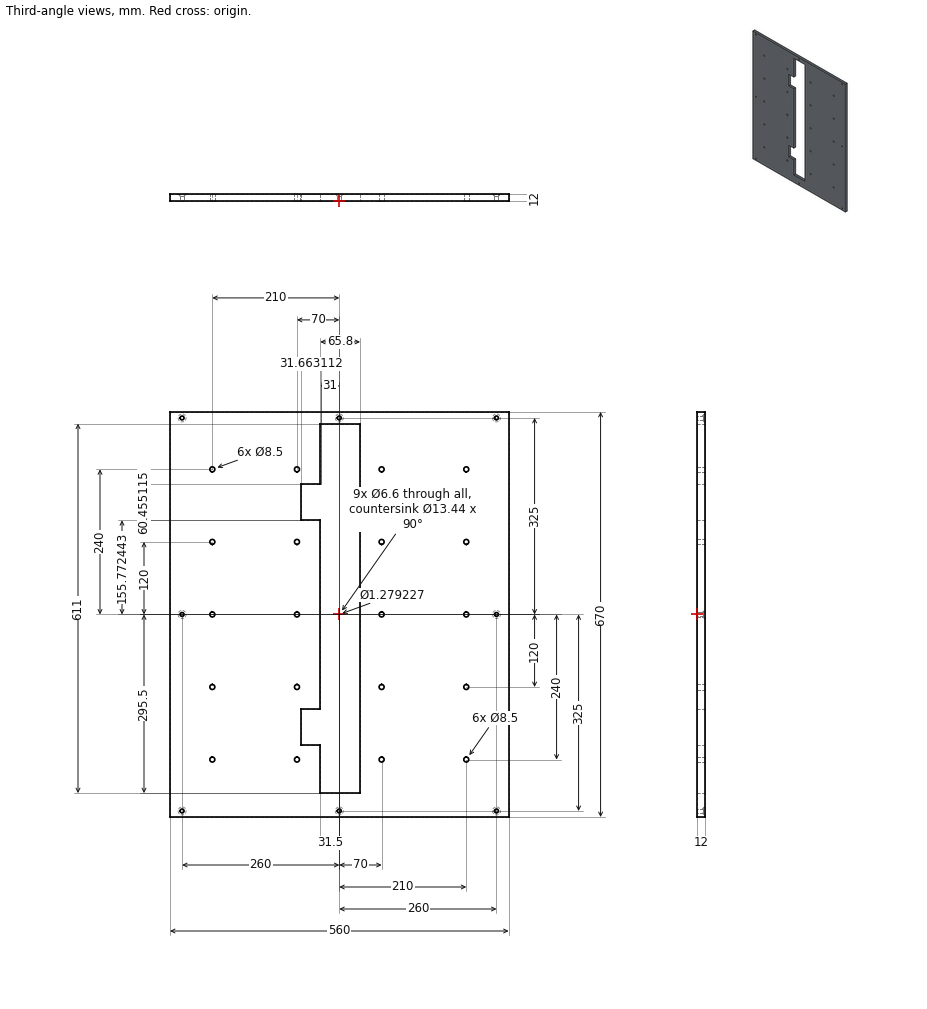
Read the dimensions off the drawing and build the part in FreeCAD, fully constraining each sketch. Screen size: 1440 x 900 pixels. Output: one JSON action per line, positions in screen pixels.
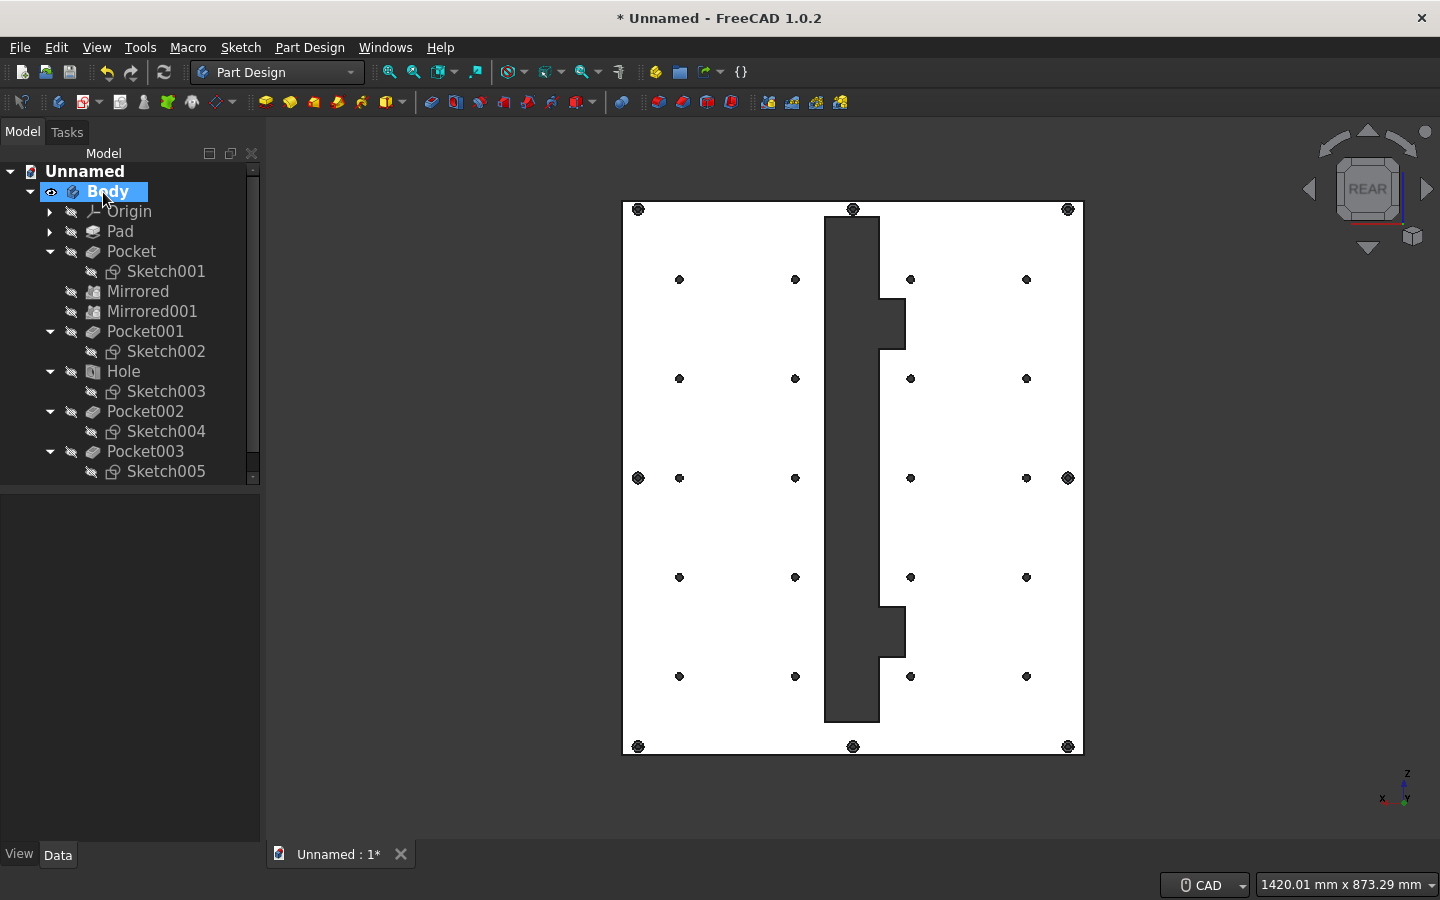
{"action": "key", "text": "0"}